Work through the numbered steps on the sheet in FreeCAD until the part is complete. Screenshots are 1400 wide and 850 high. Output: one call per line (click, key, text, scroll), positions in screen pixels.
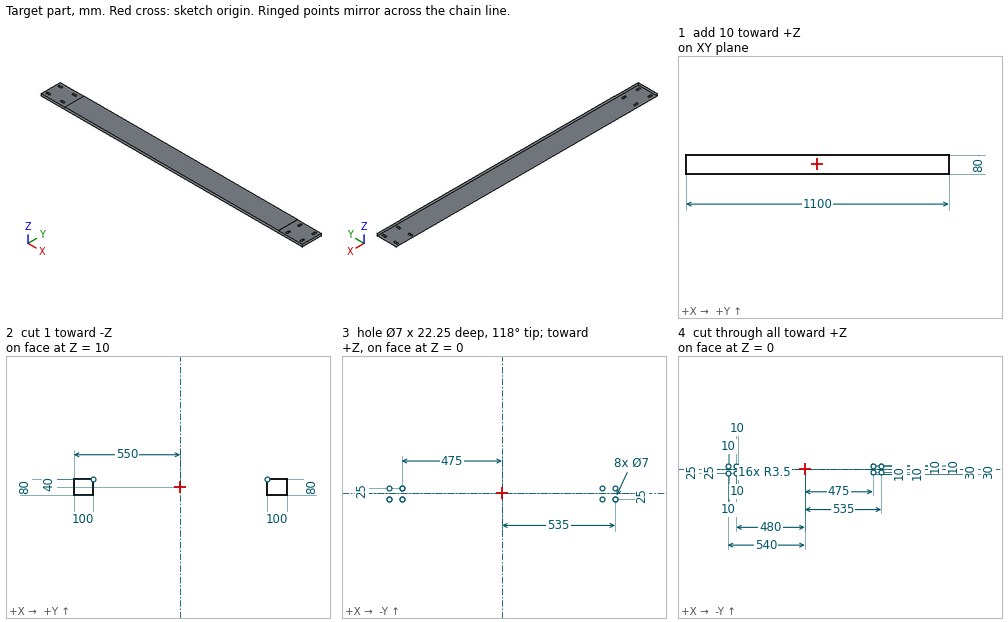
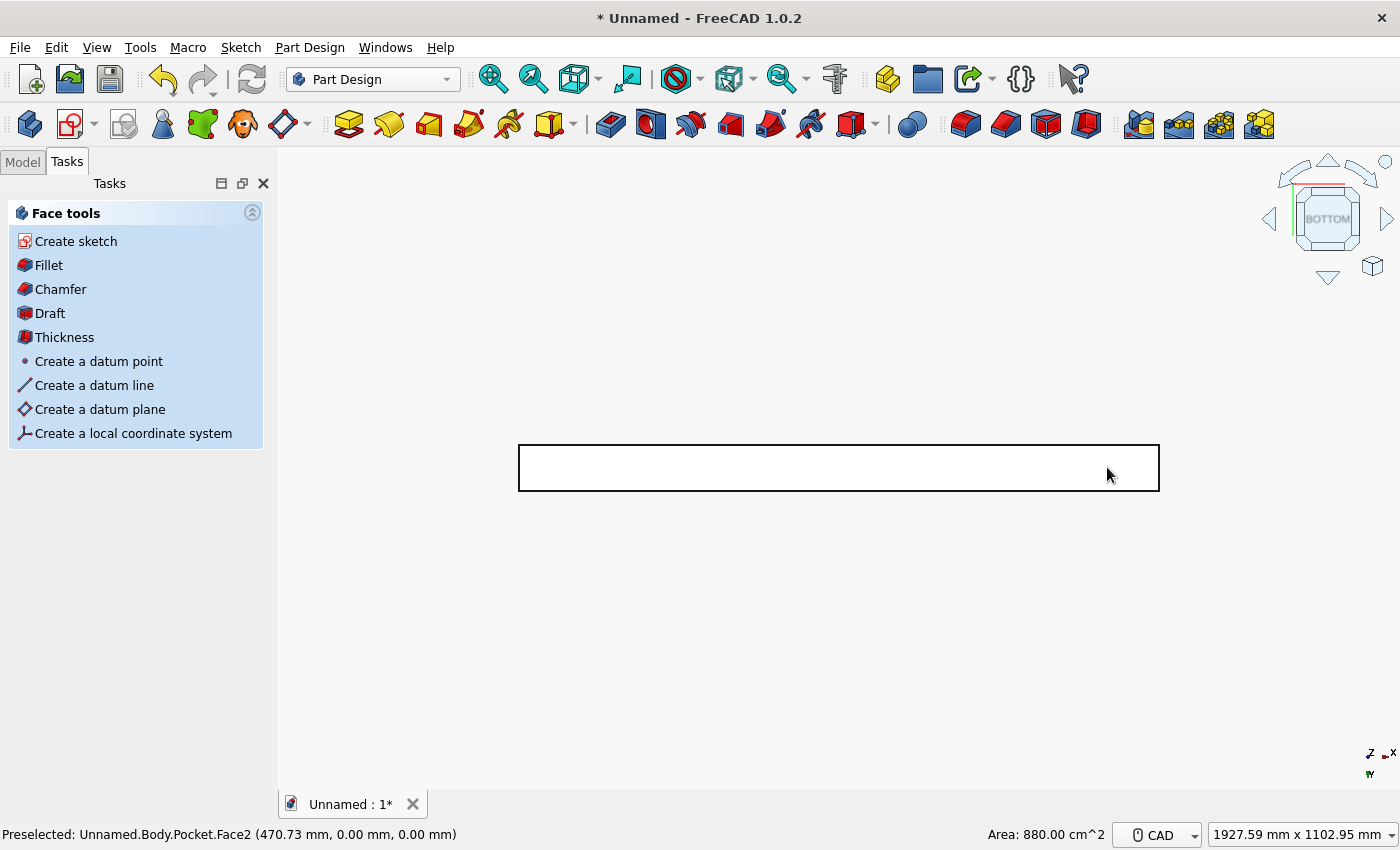
click(70, 124)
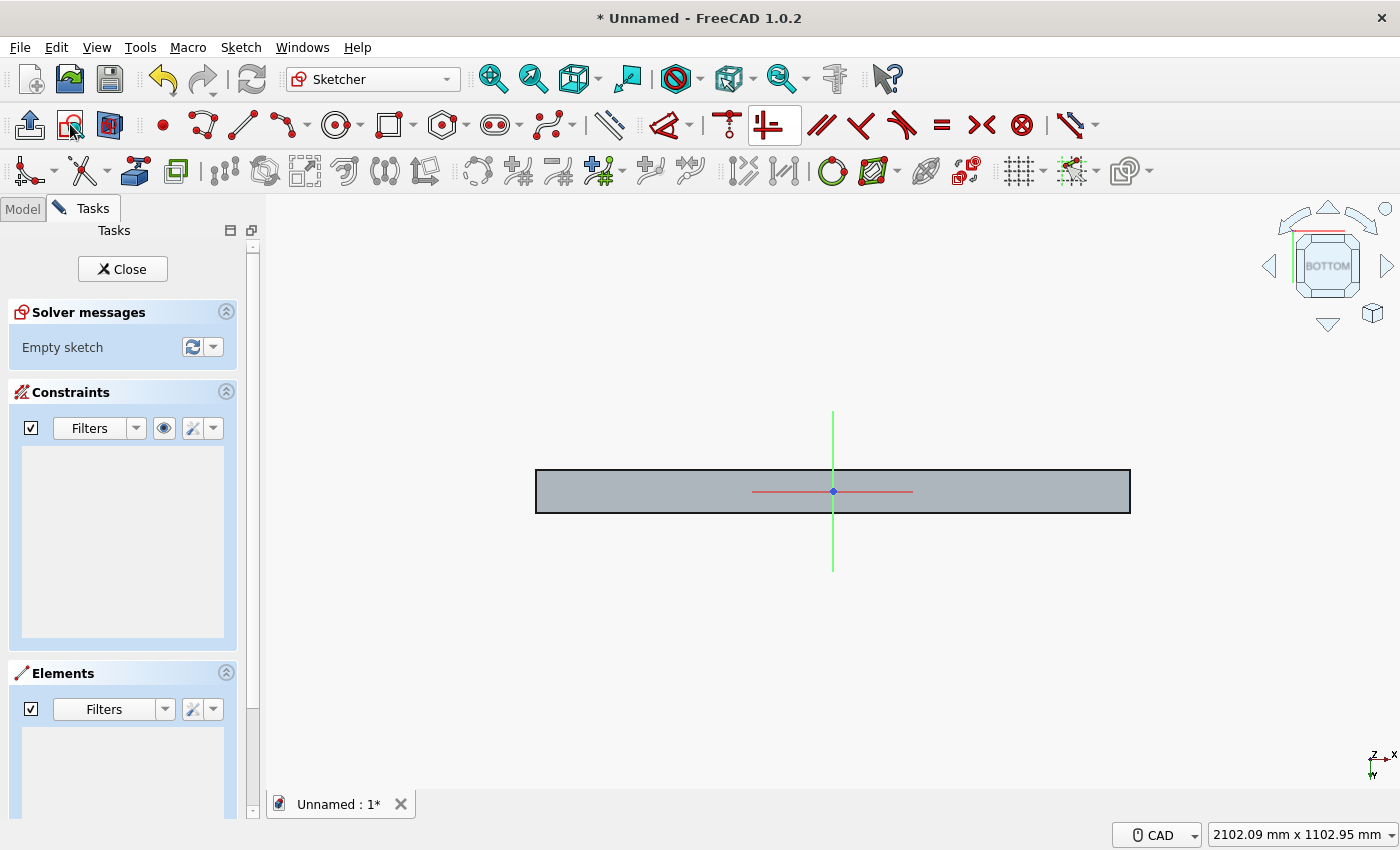
click(336, 126)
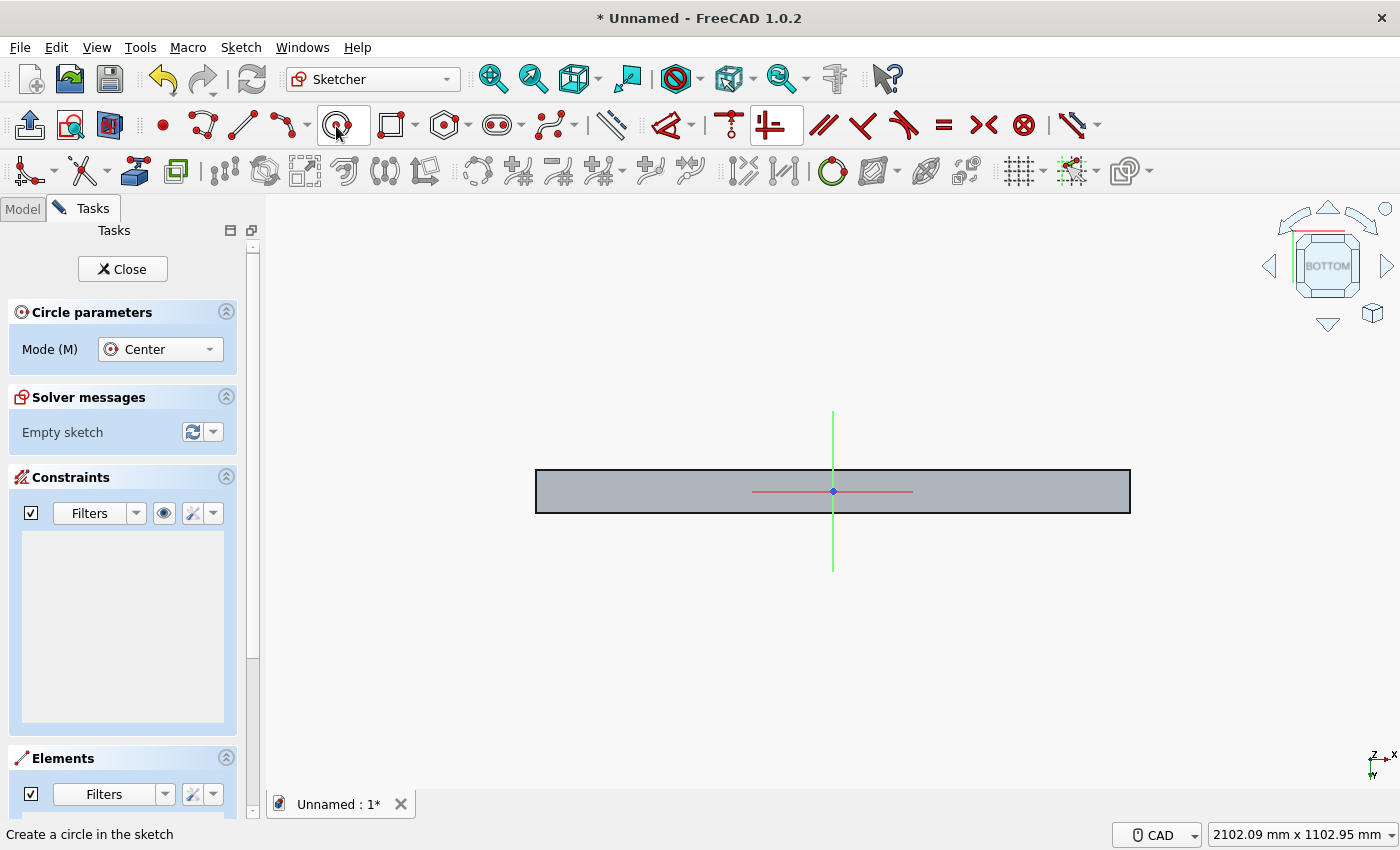
scroll(1122, 505, up, 13)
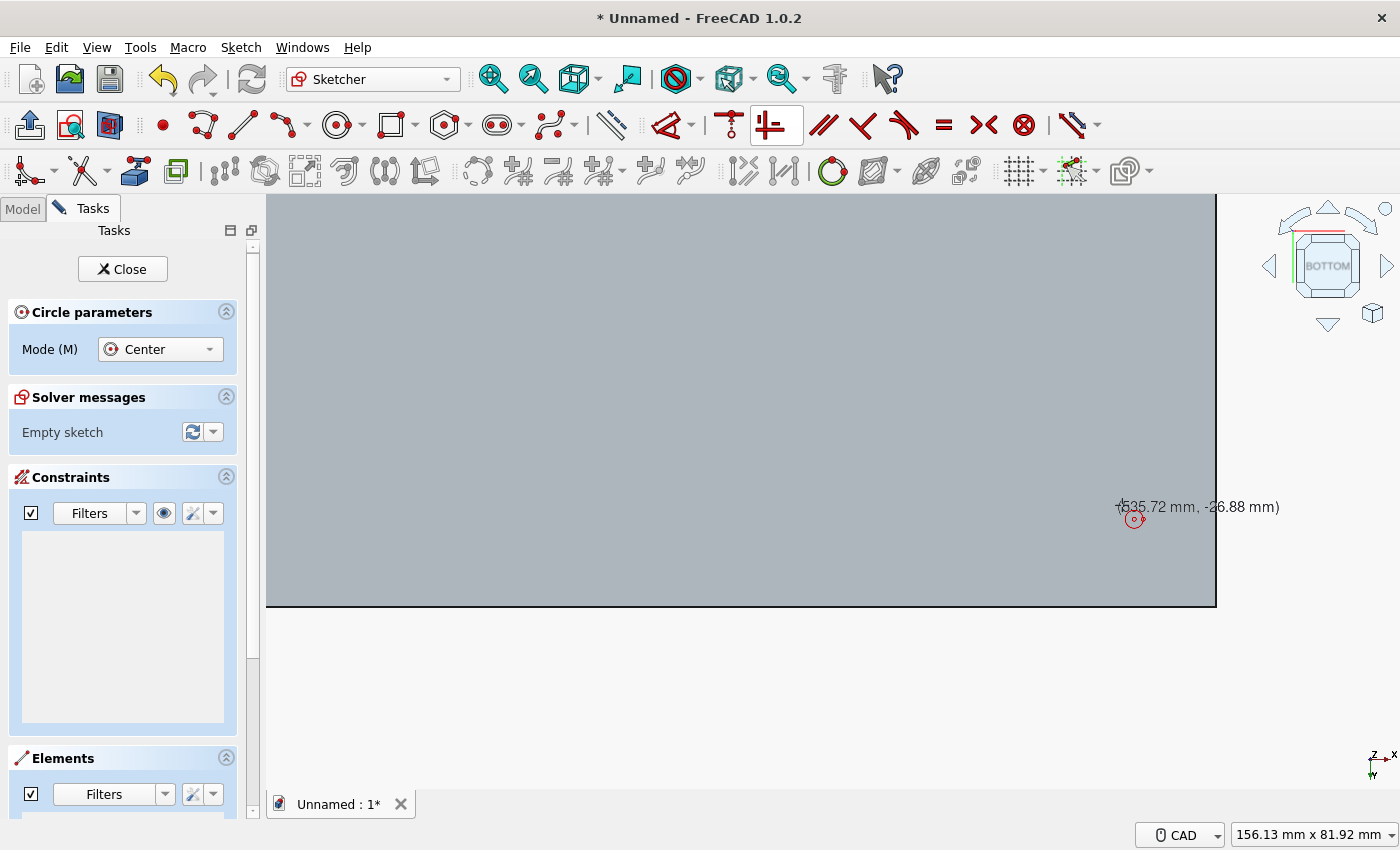
scroll(1118, 509, down, 12)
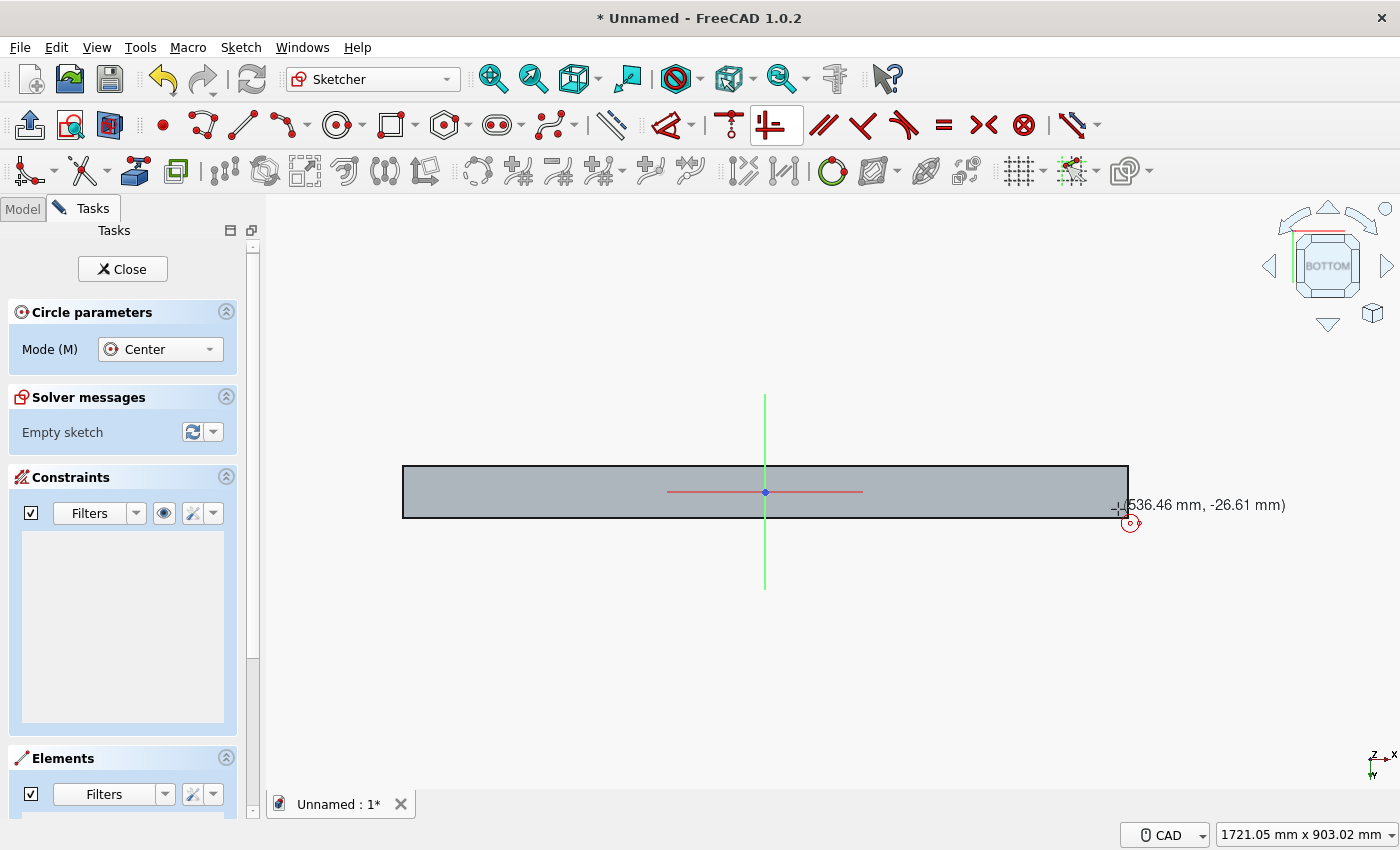
click(1118, 509)
move(1119, 507)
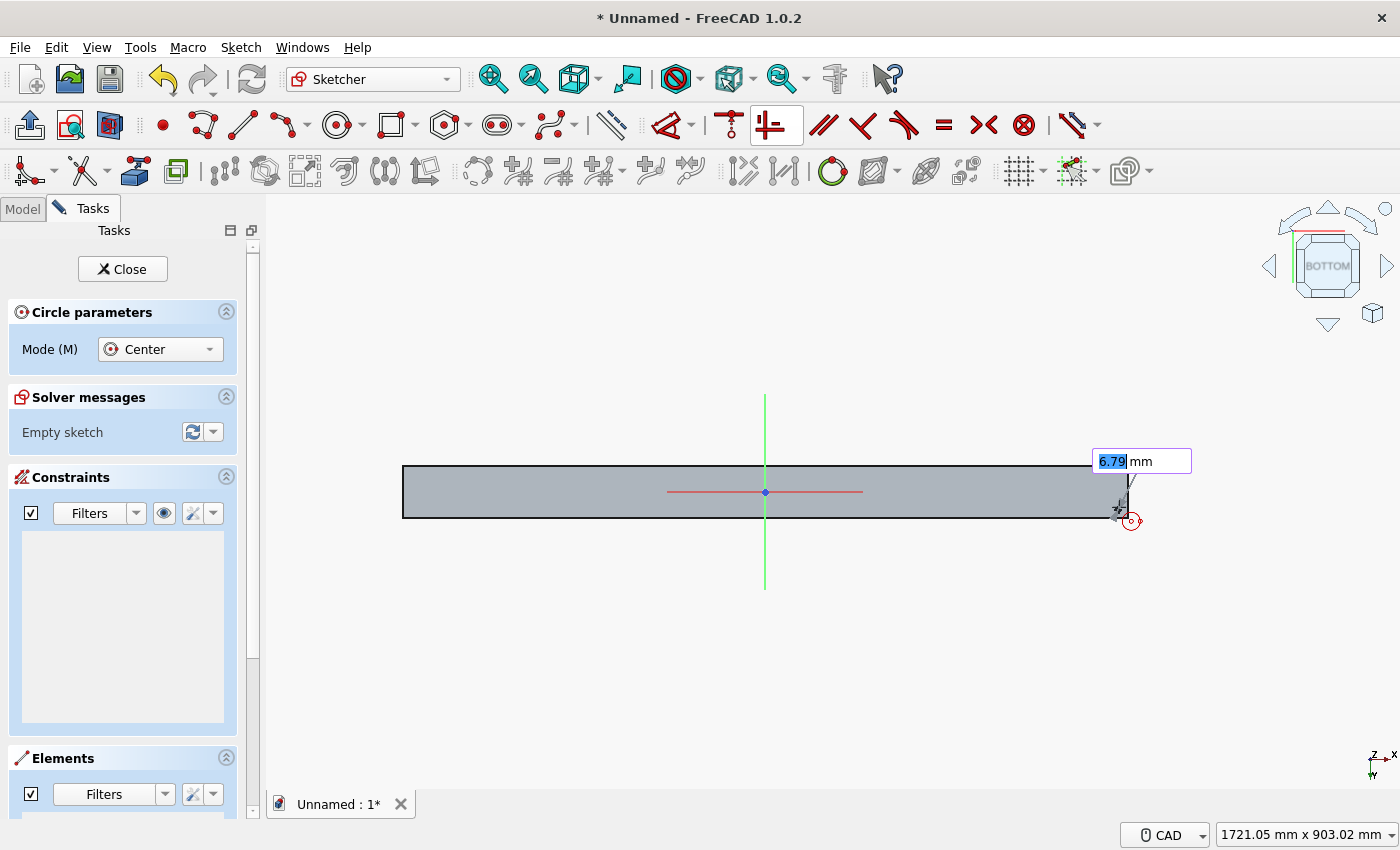
text(7)
key(Return)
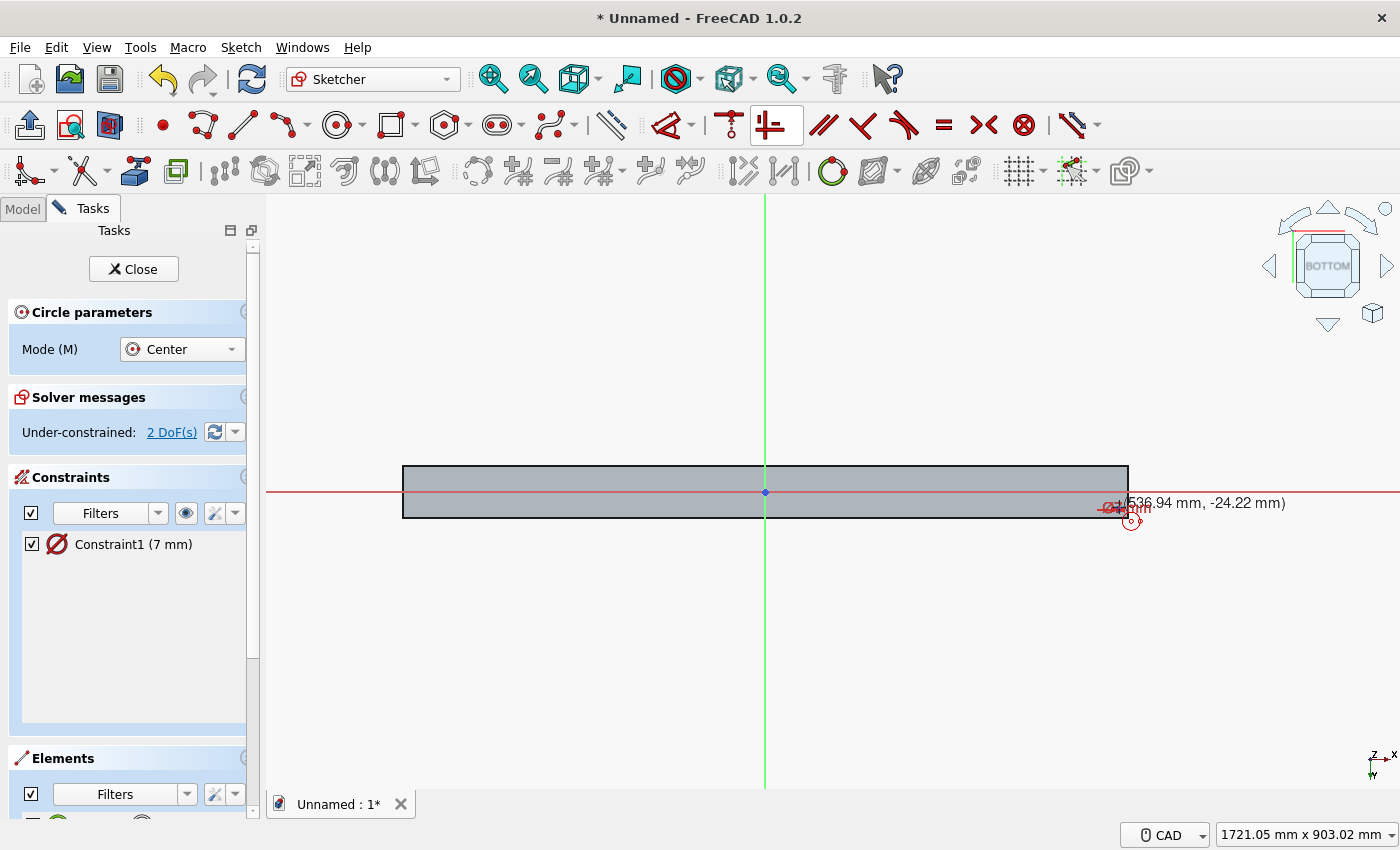
scroll(452, 476, up, 12)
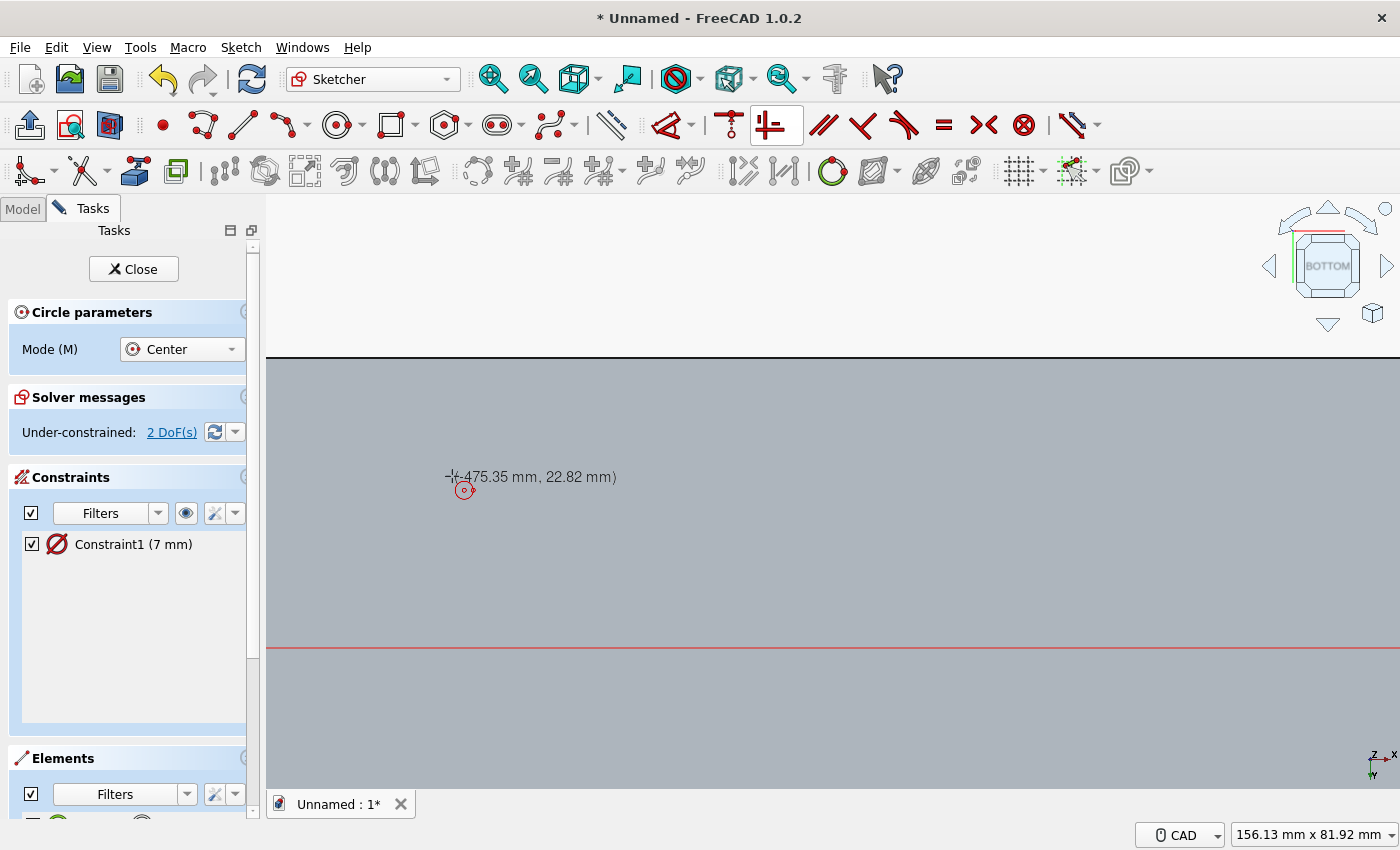
scroll(451, 476, down, 12)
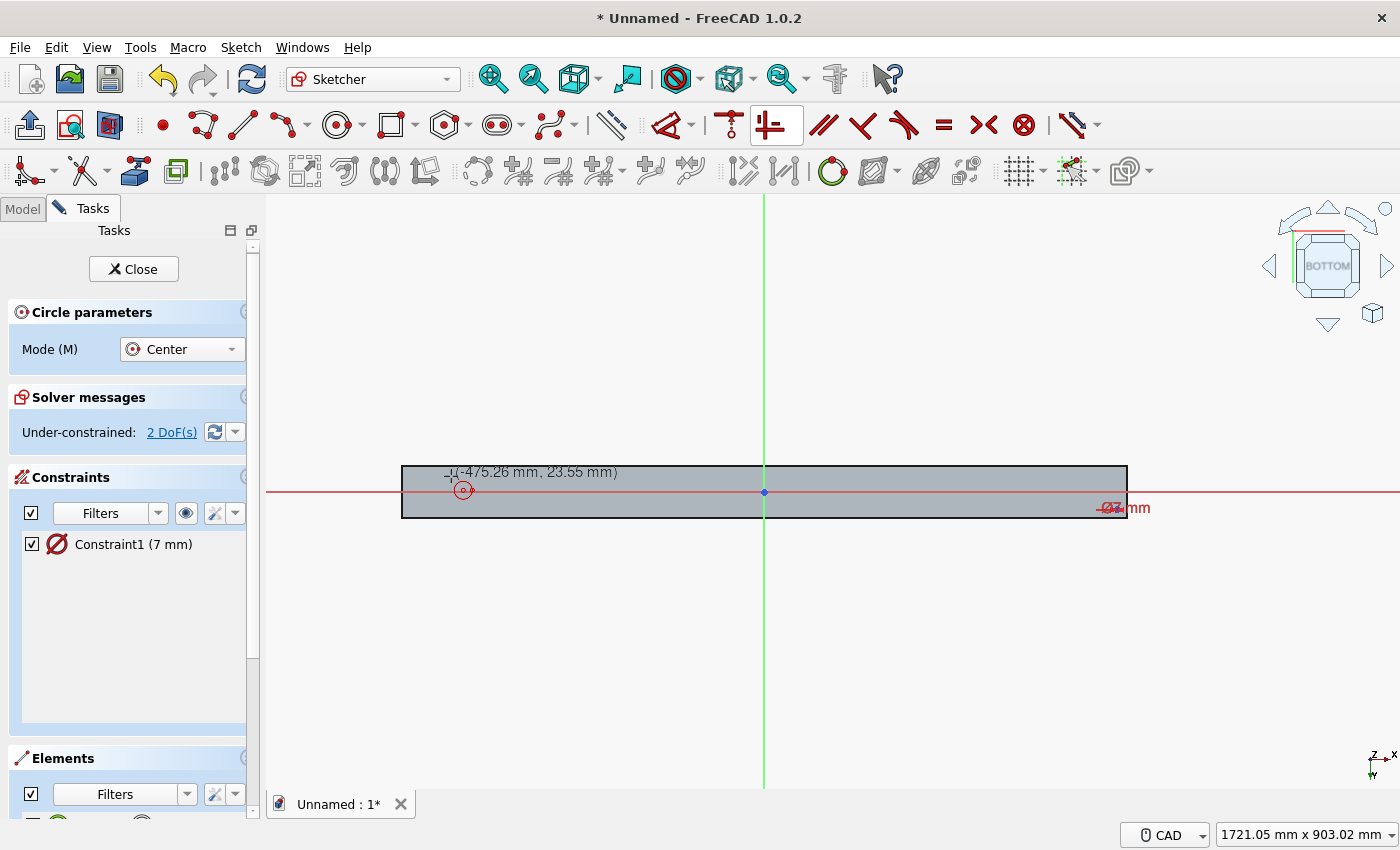
click(451, 476)
move(453, 474)